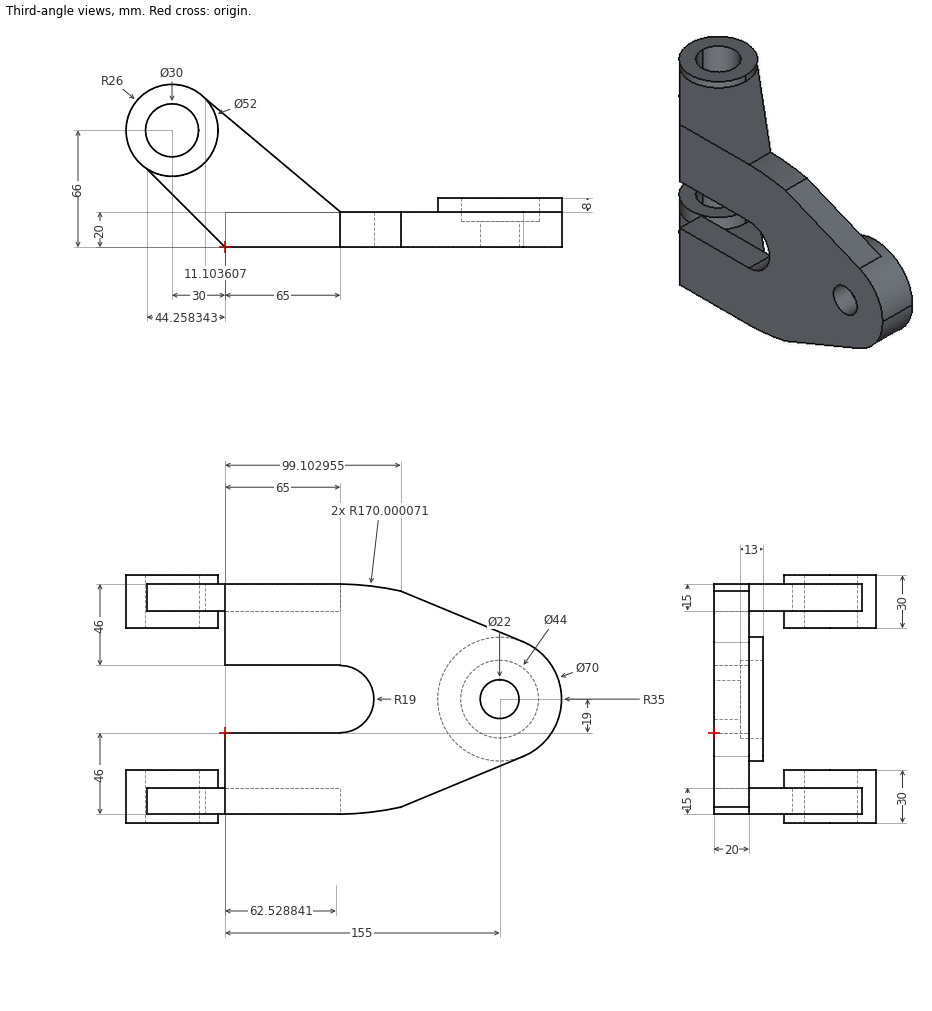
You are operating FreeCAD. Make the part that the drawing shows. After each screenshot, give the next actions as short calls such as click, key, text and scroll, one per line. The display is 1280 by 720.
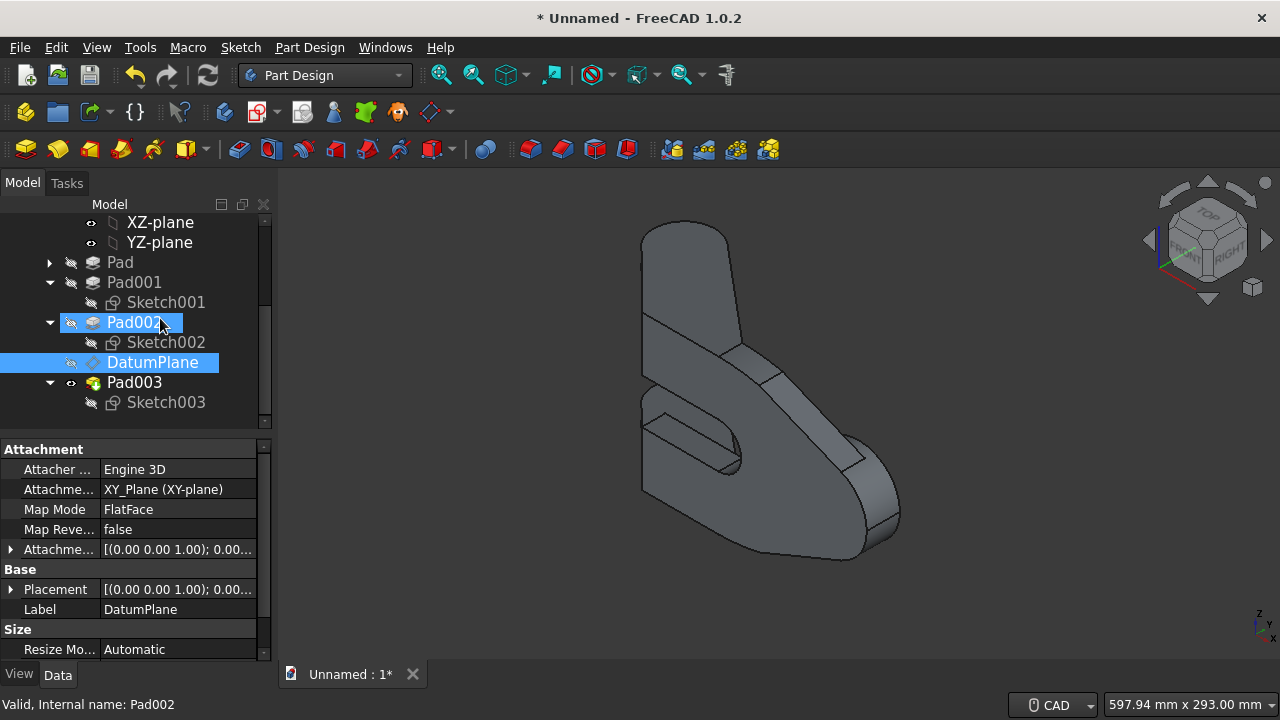
scroll(160, 318, up, 15)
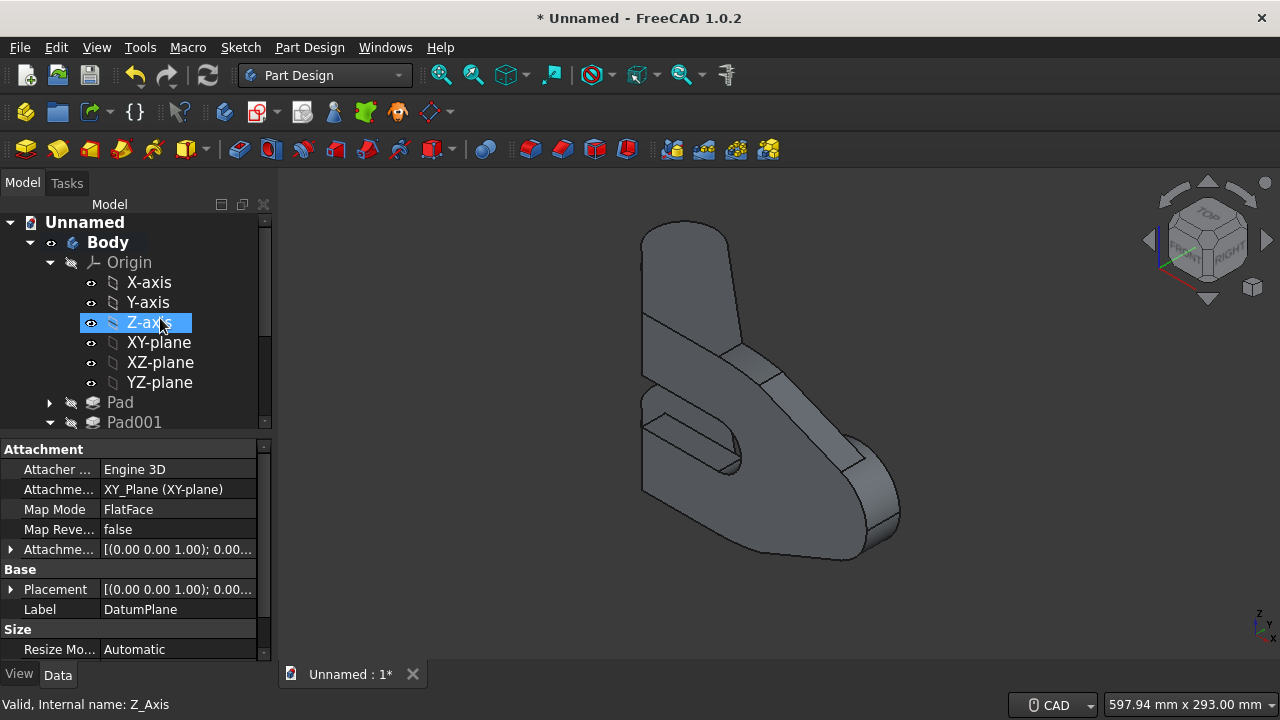
click(136, 343)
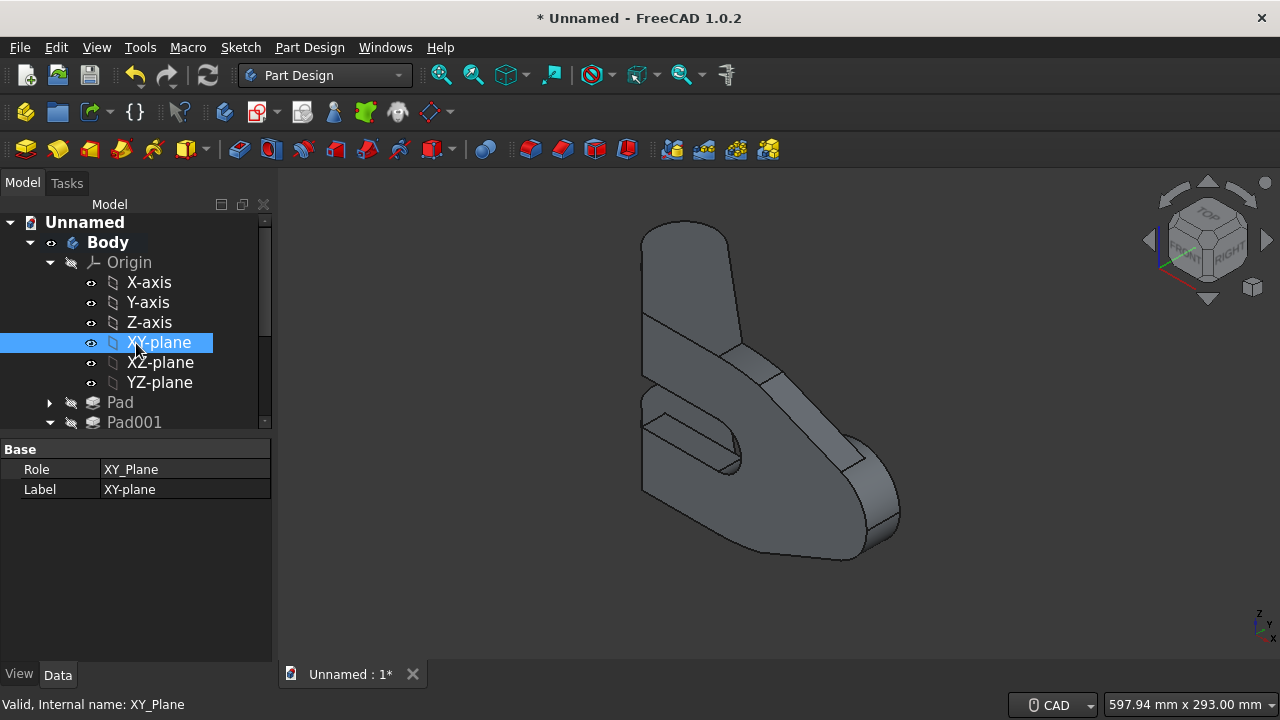
click(430, 112)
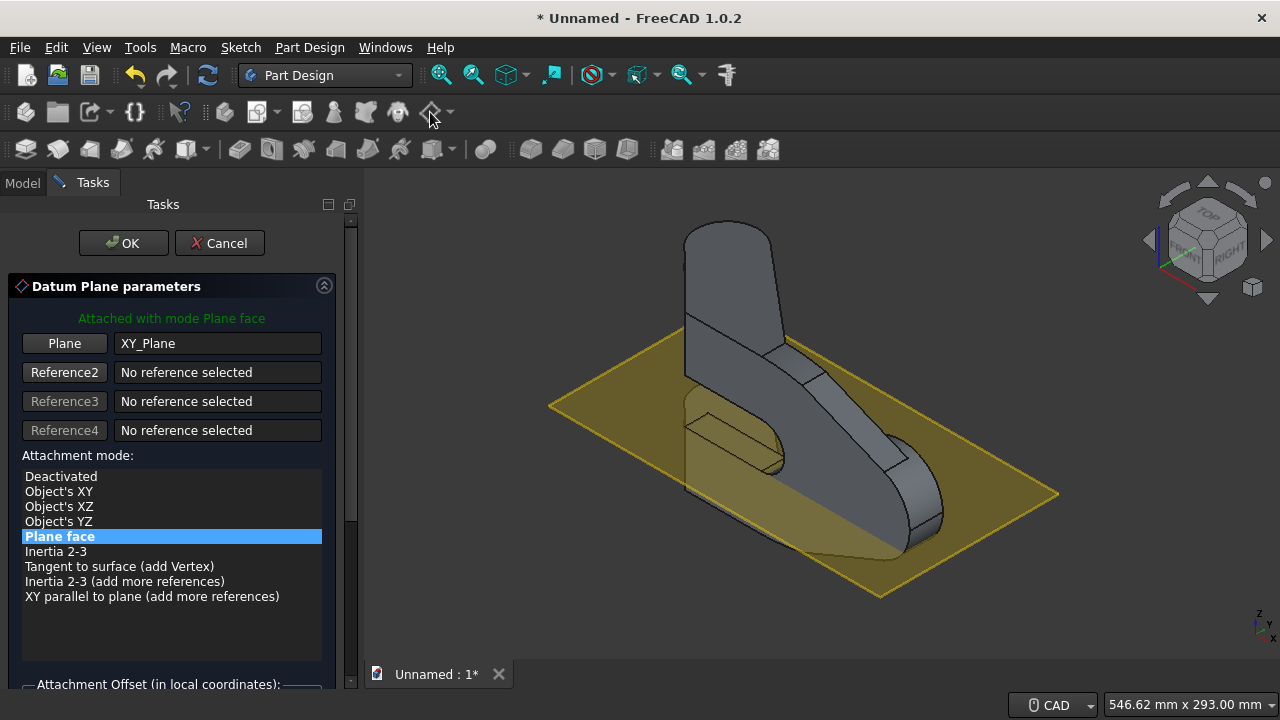
scroll(351, 451, down, 3)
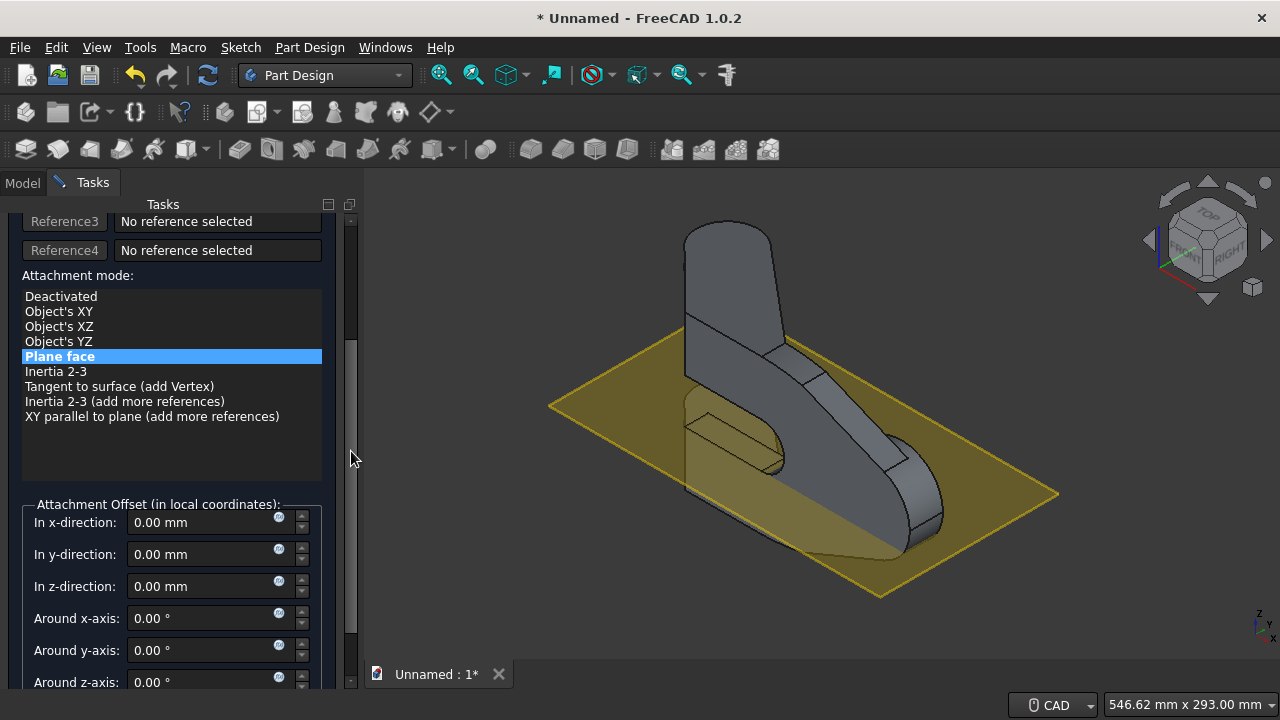
triple_click(210, 586)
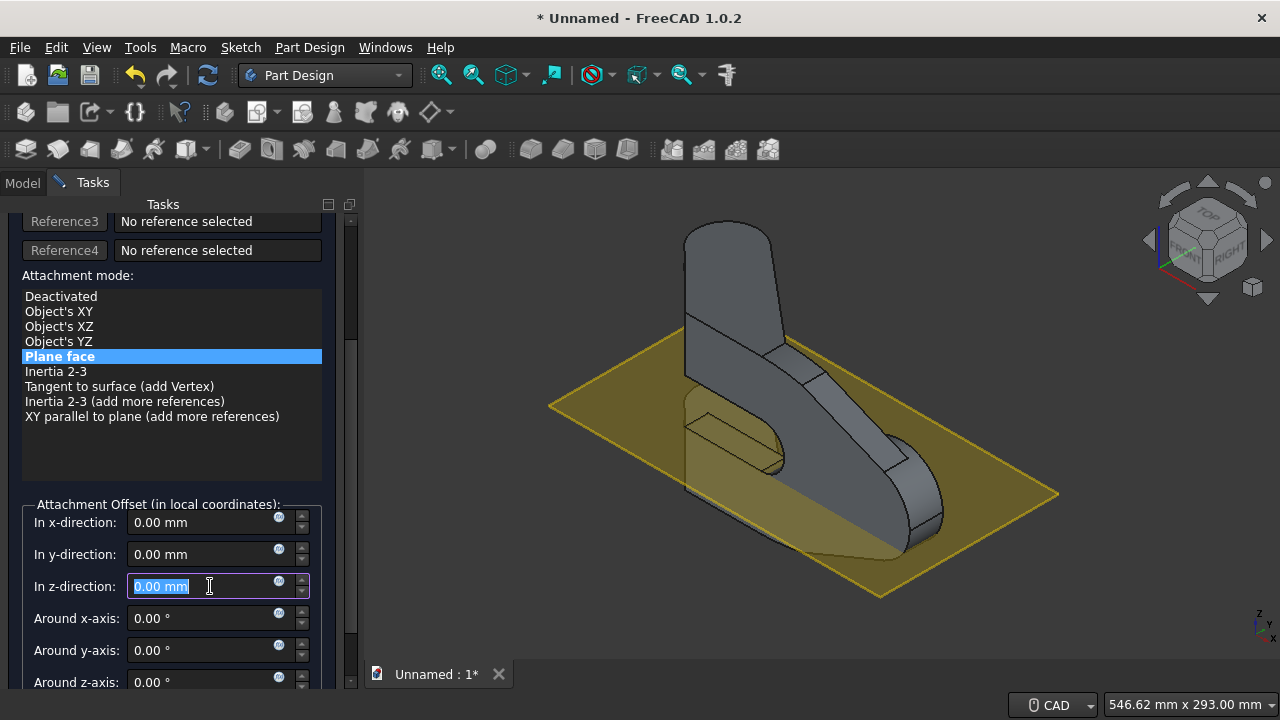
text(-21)
key(Tab)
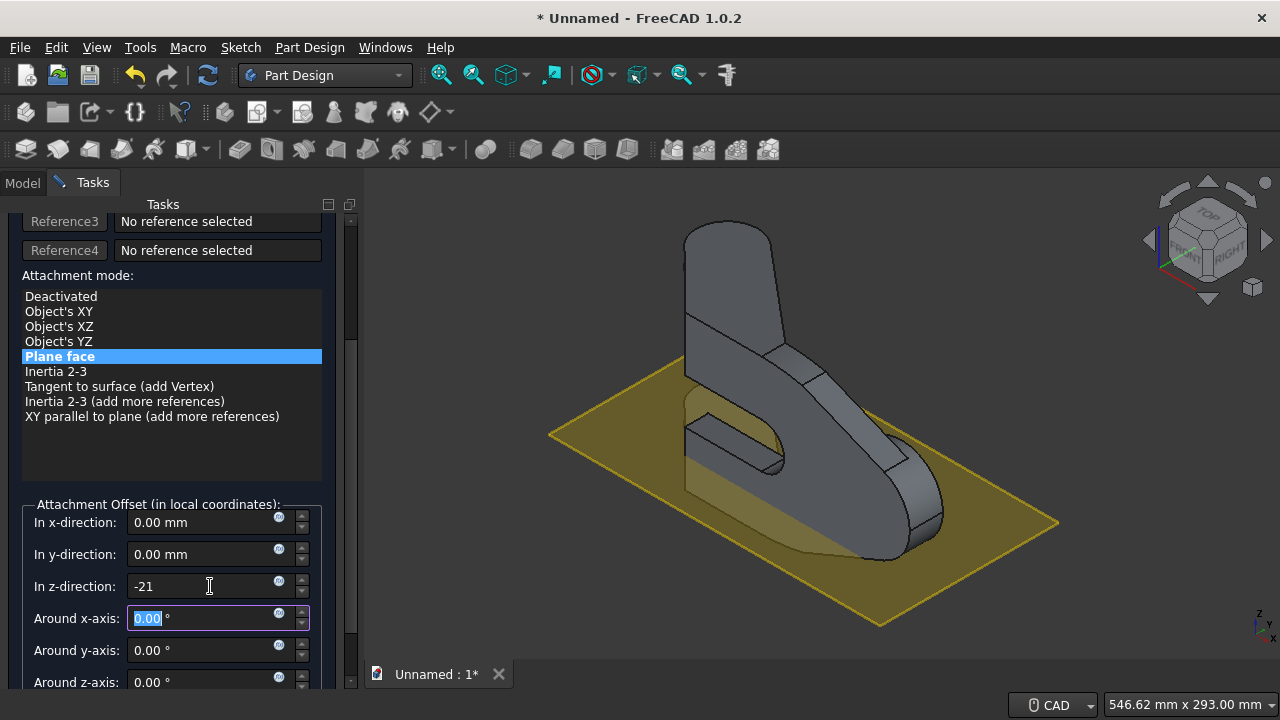
scroll(351, 451, up, 4)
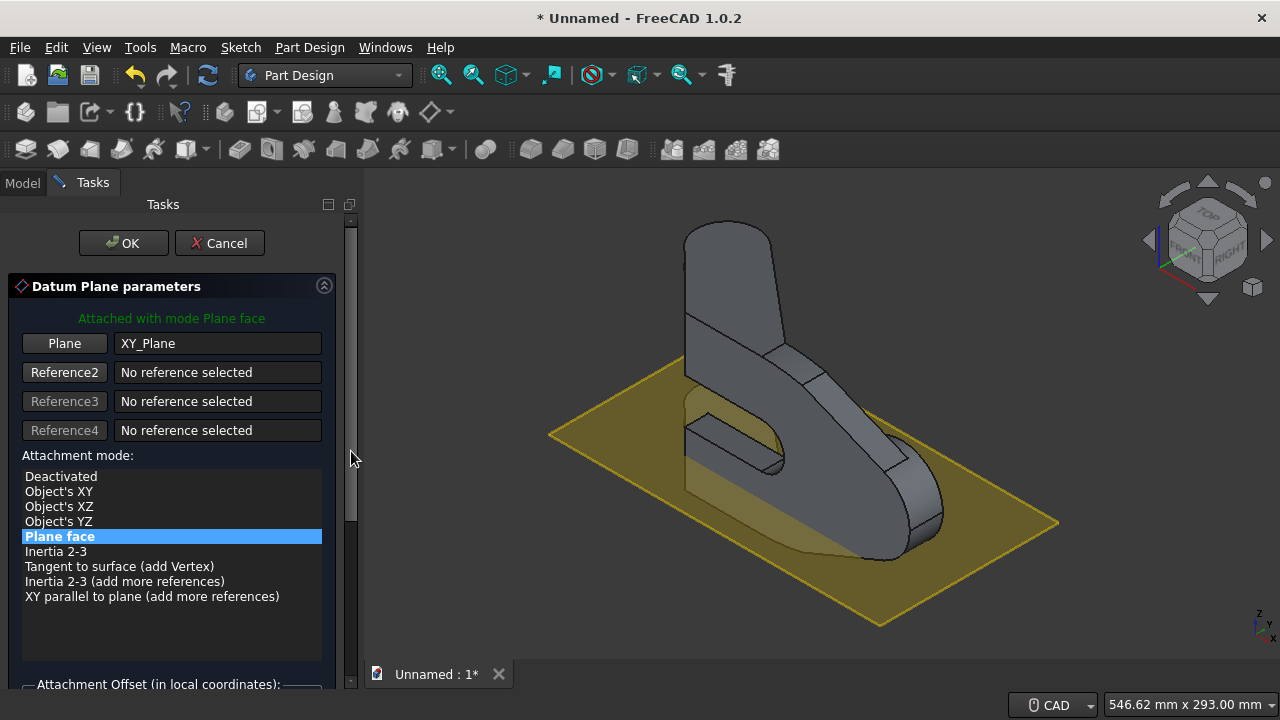
click(124, 243)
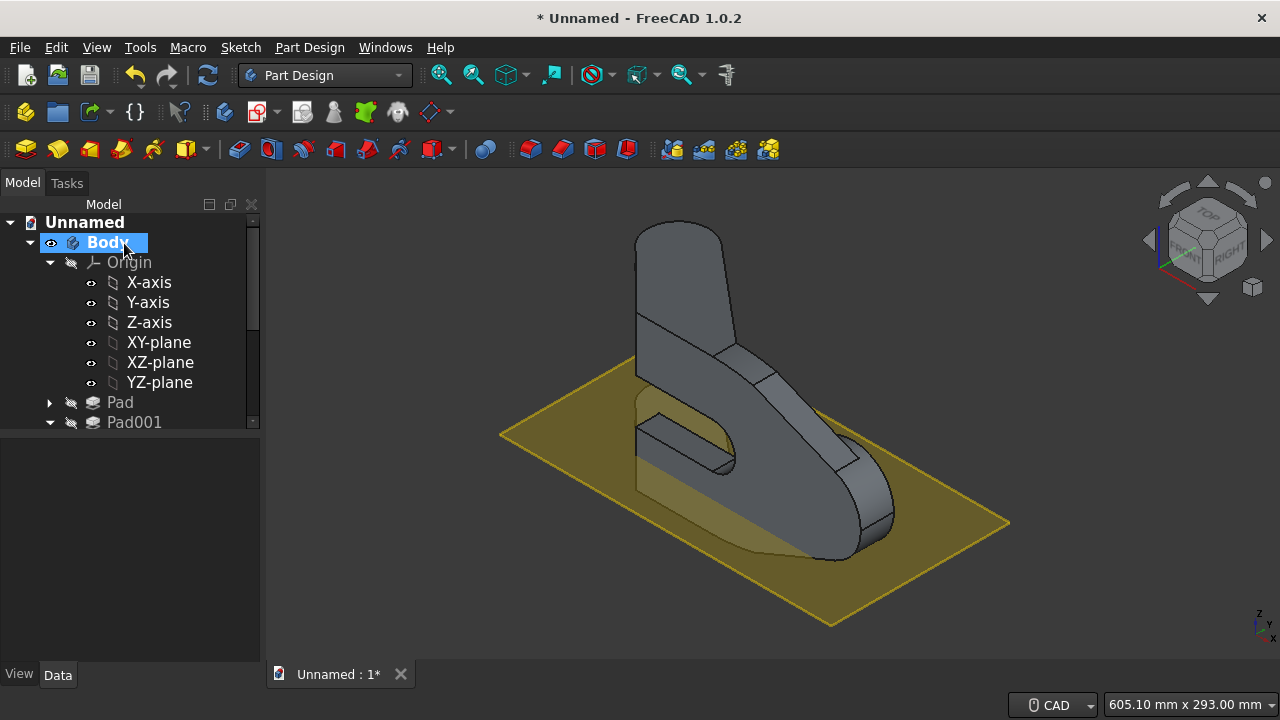
scroll(100, 318, down, 3)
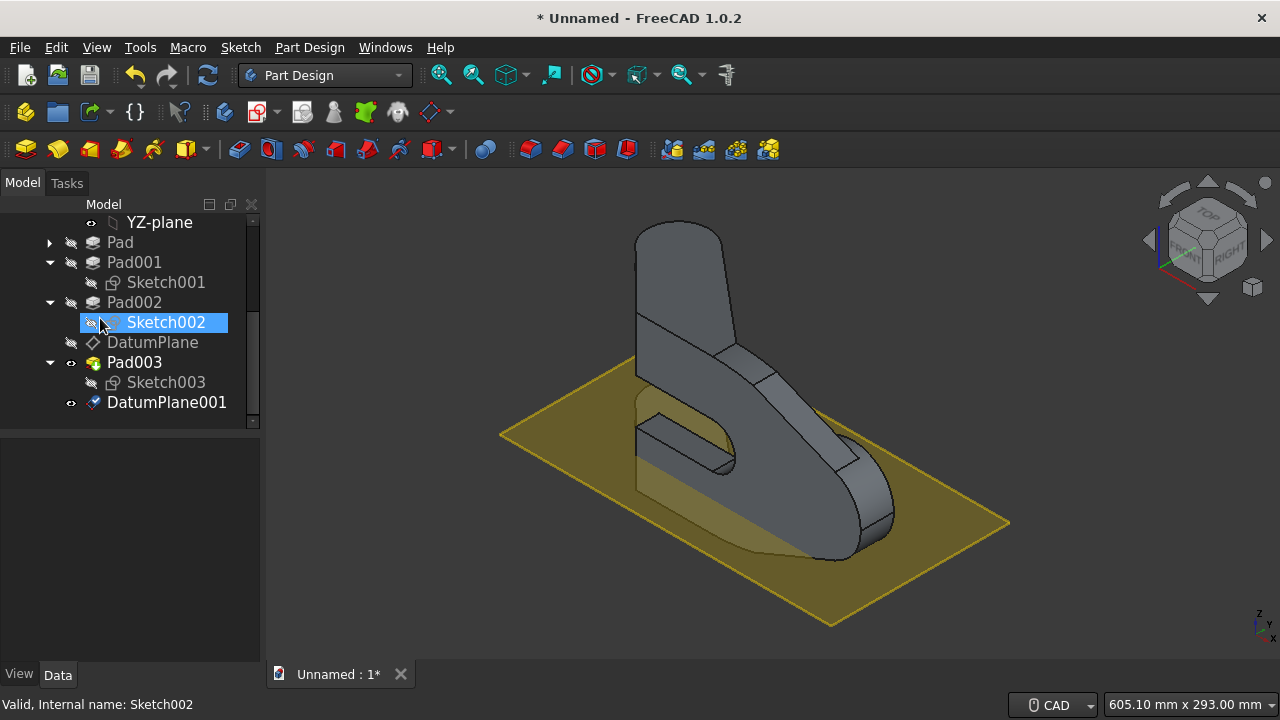
click(116, 403)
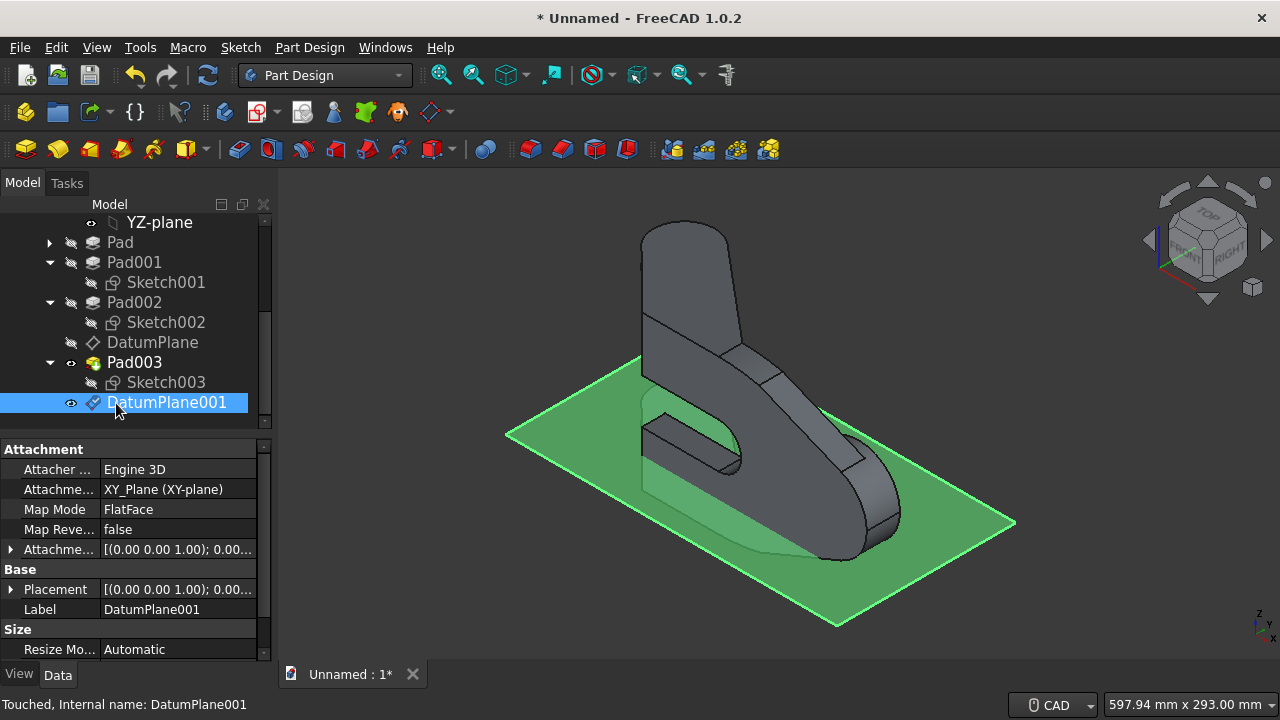
click(258, 112)